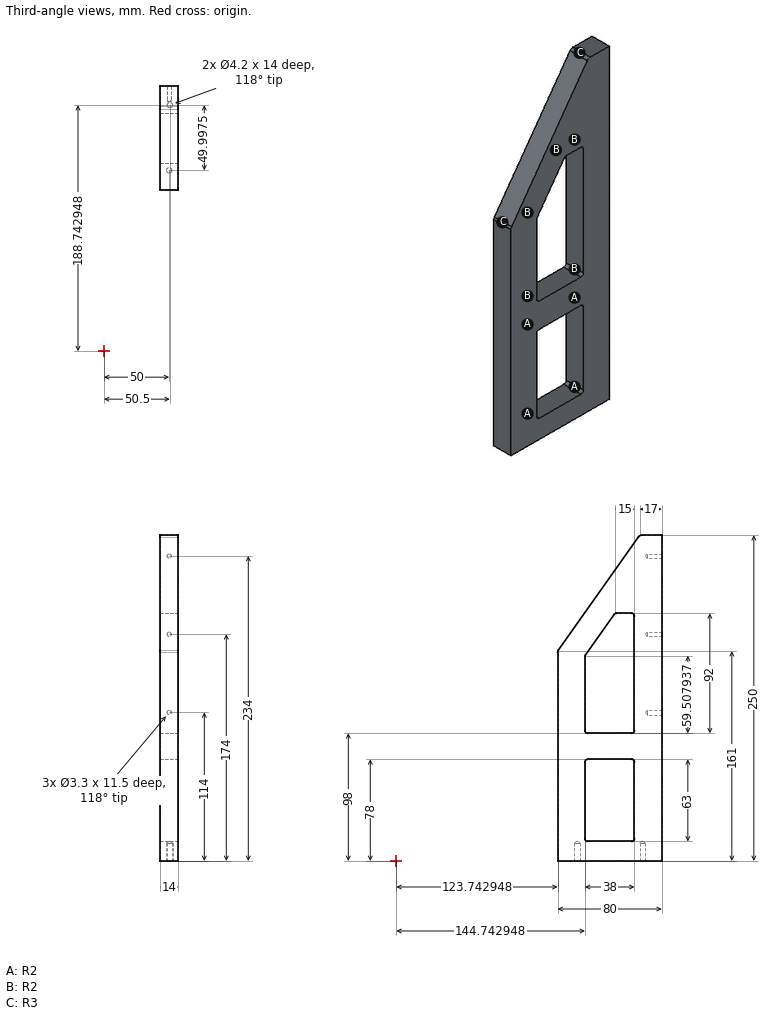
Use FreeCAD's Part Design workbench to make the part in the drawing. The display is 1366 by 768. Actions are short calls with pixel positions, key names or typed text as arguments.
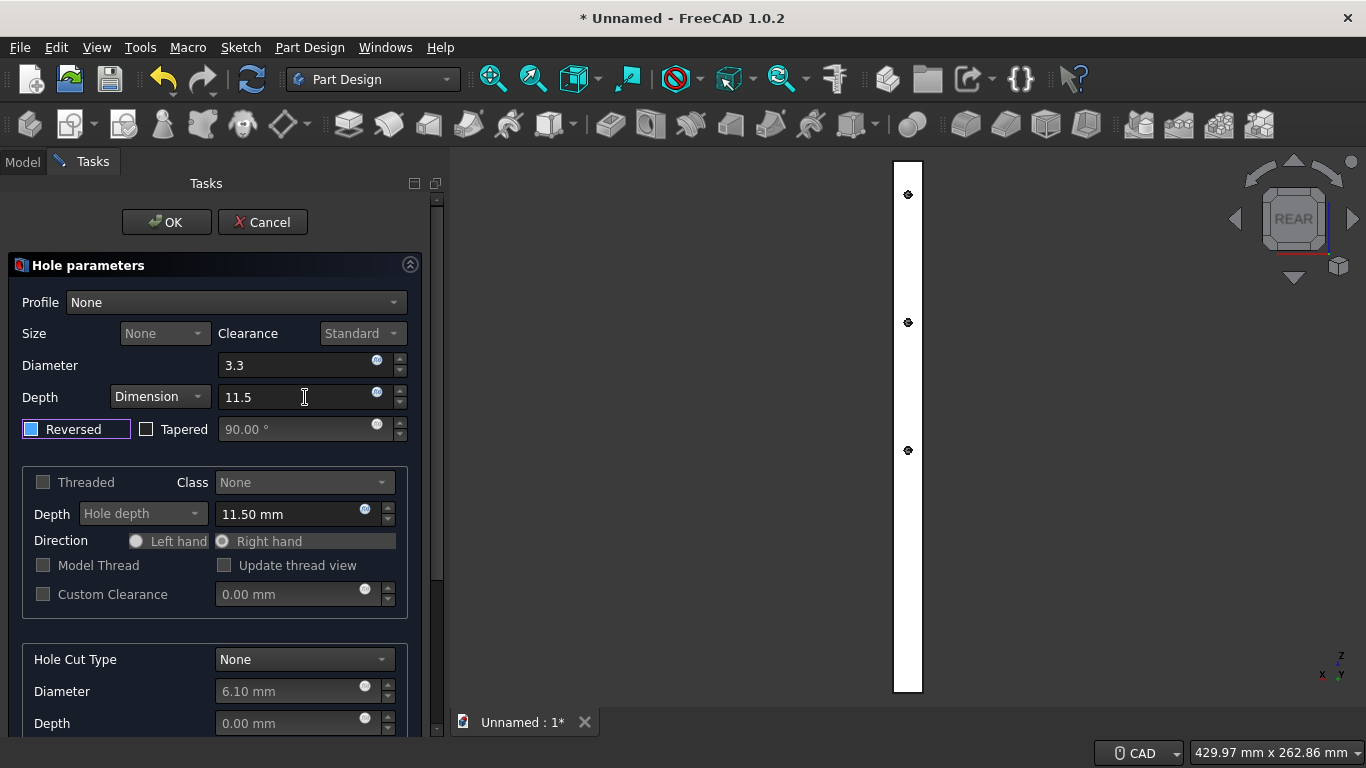
click(167, 222)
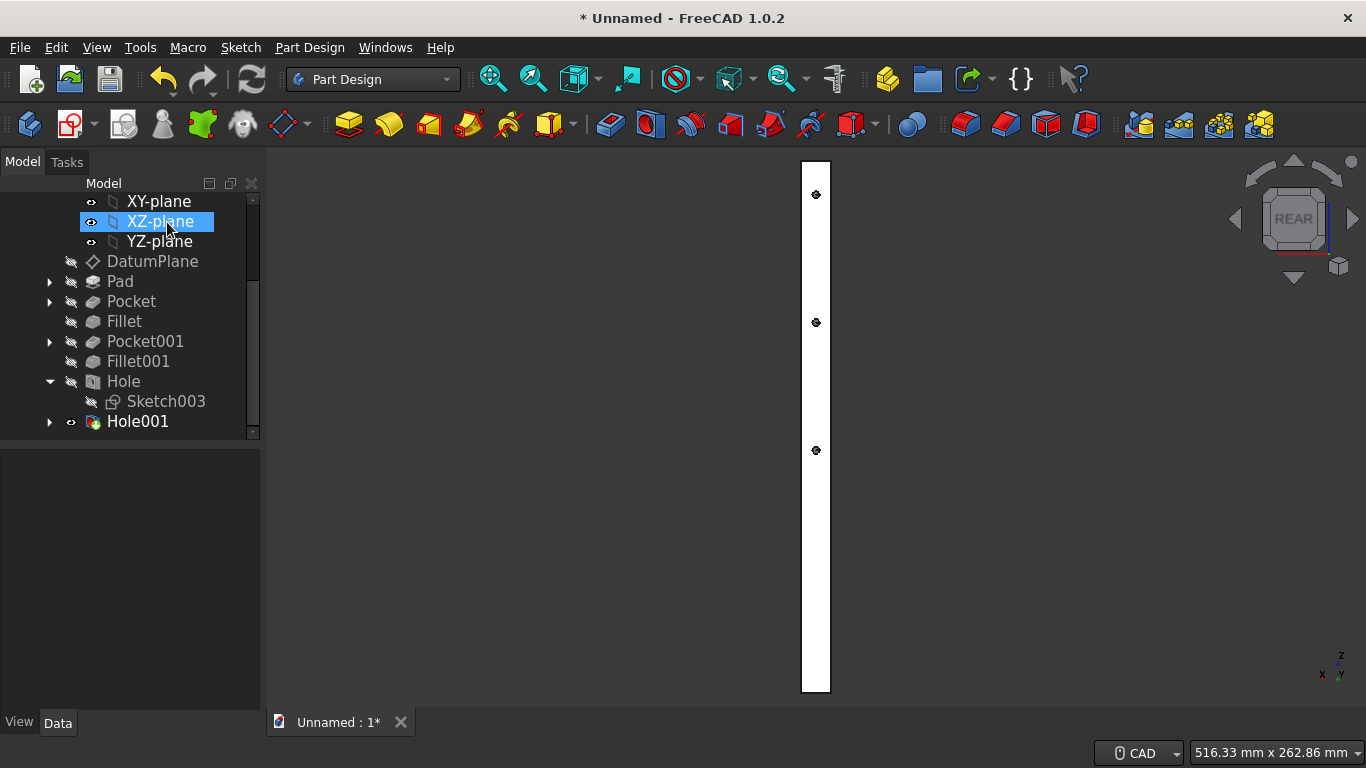
key(0)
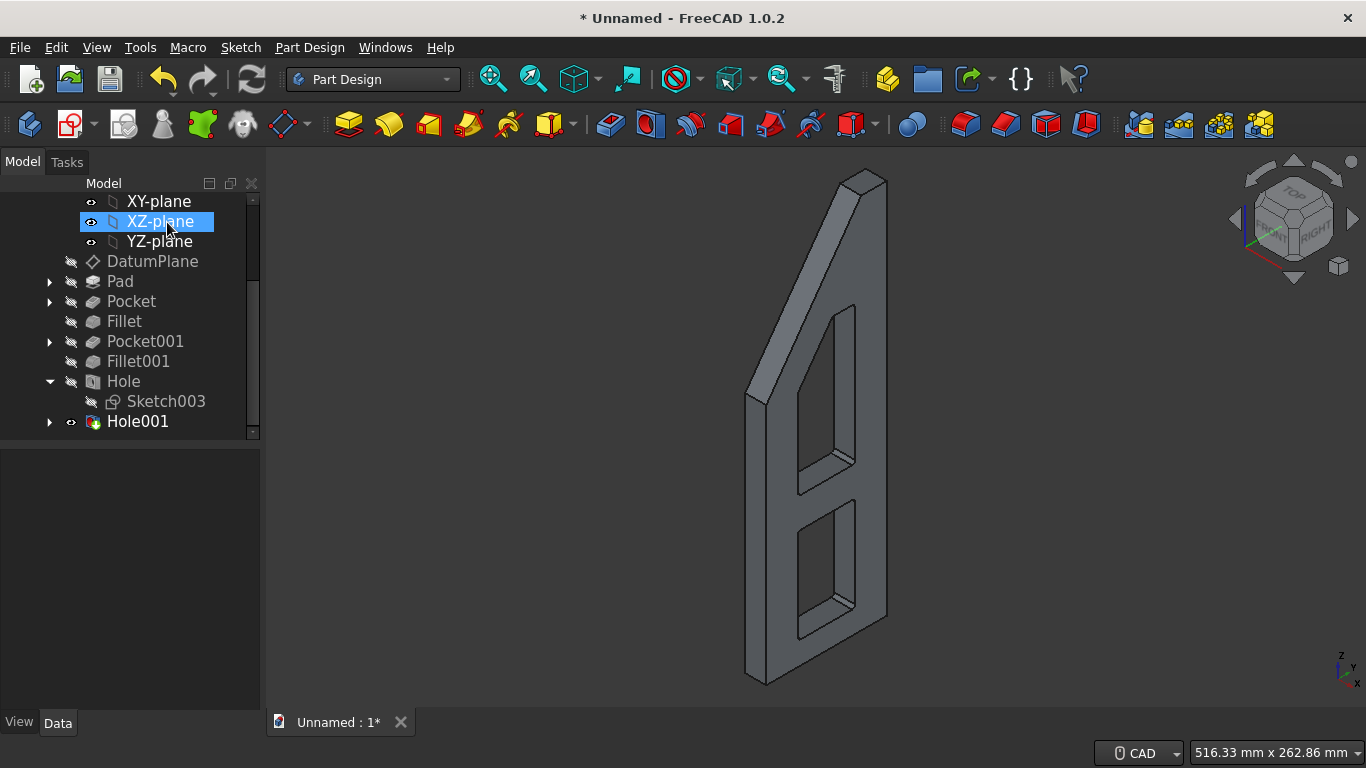
click(851, 189)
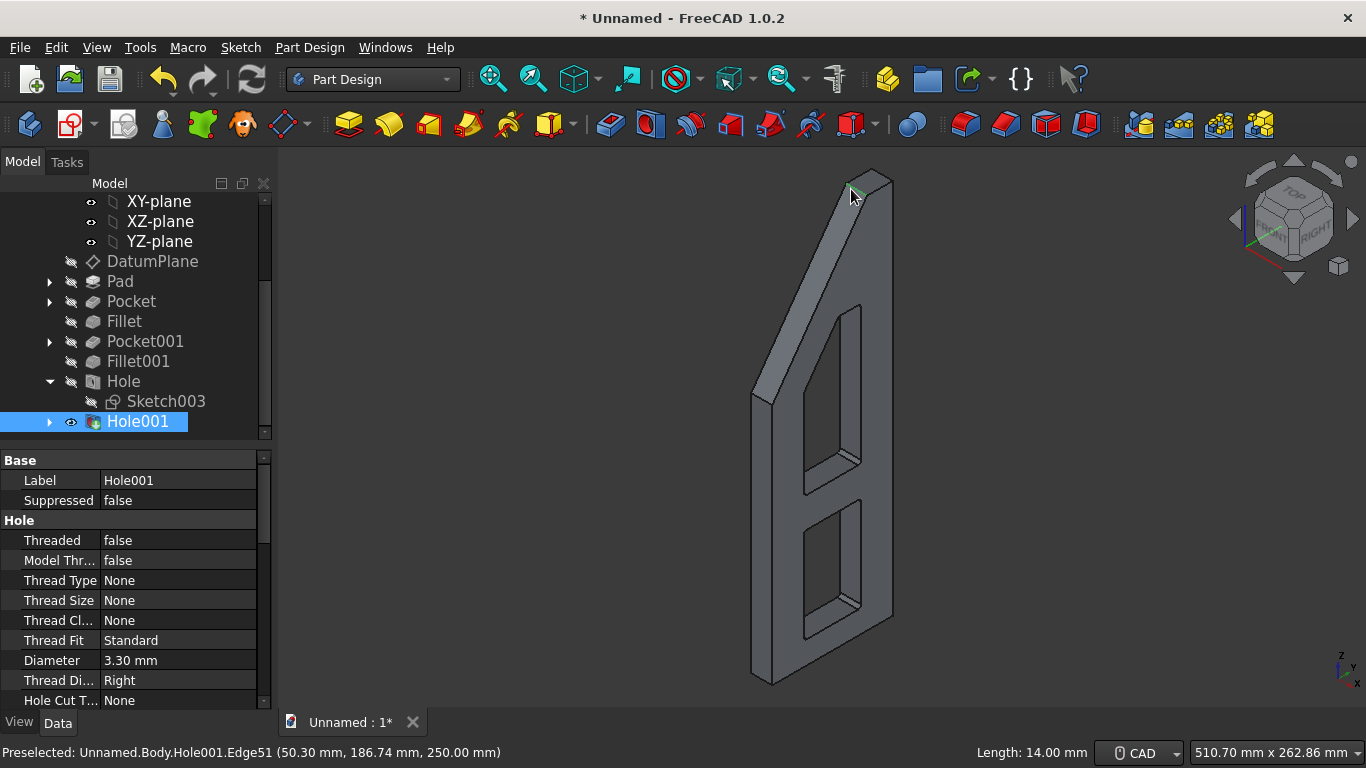
key(2)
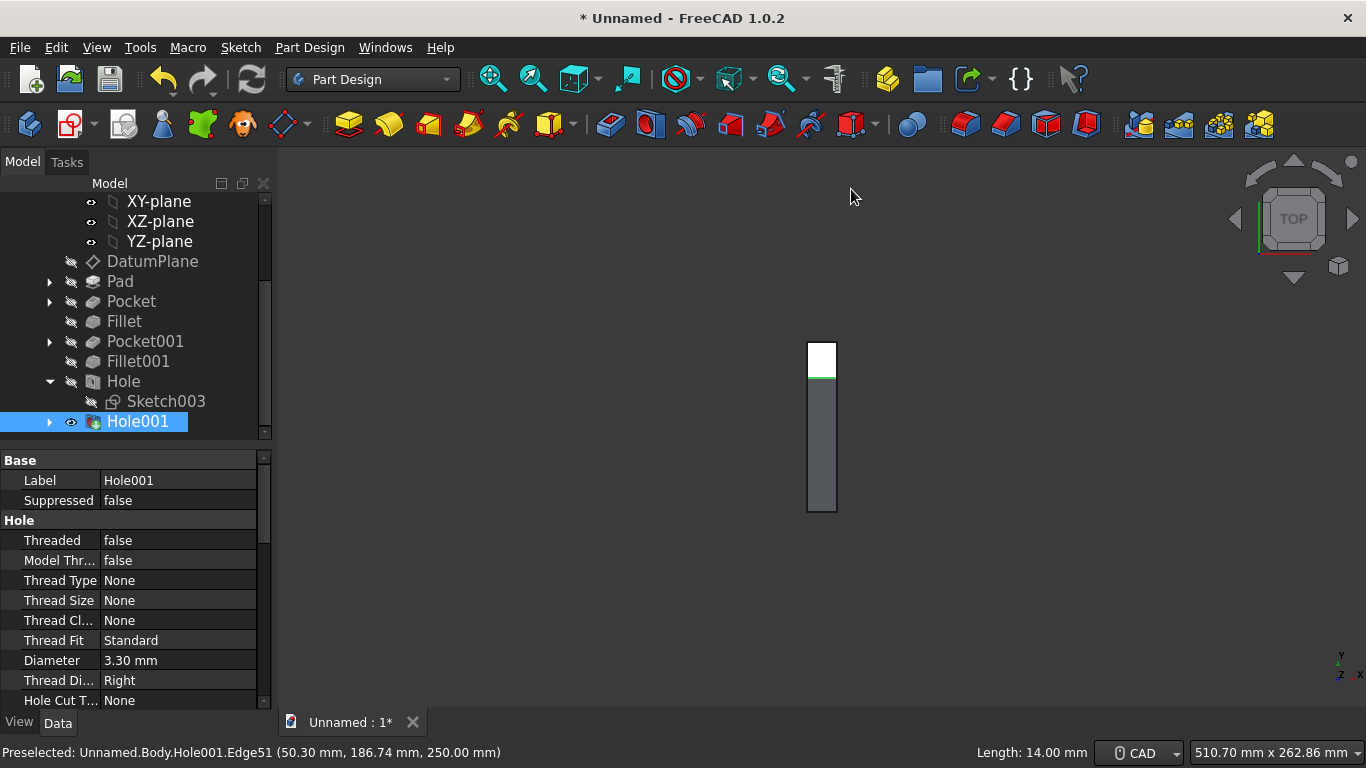
click(494, 80)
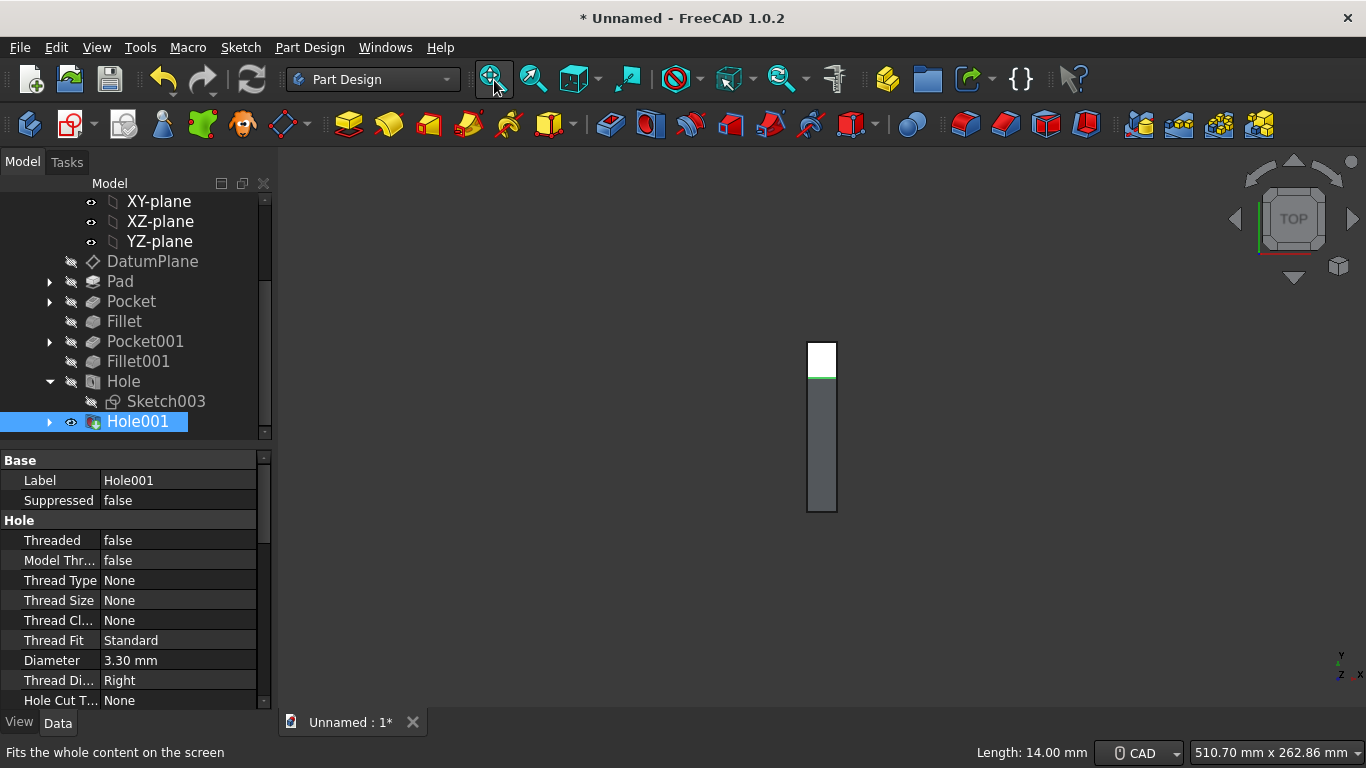
key(1)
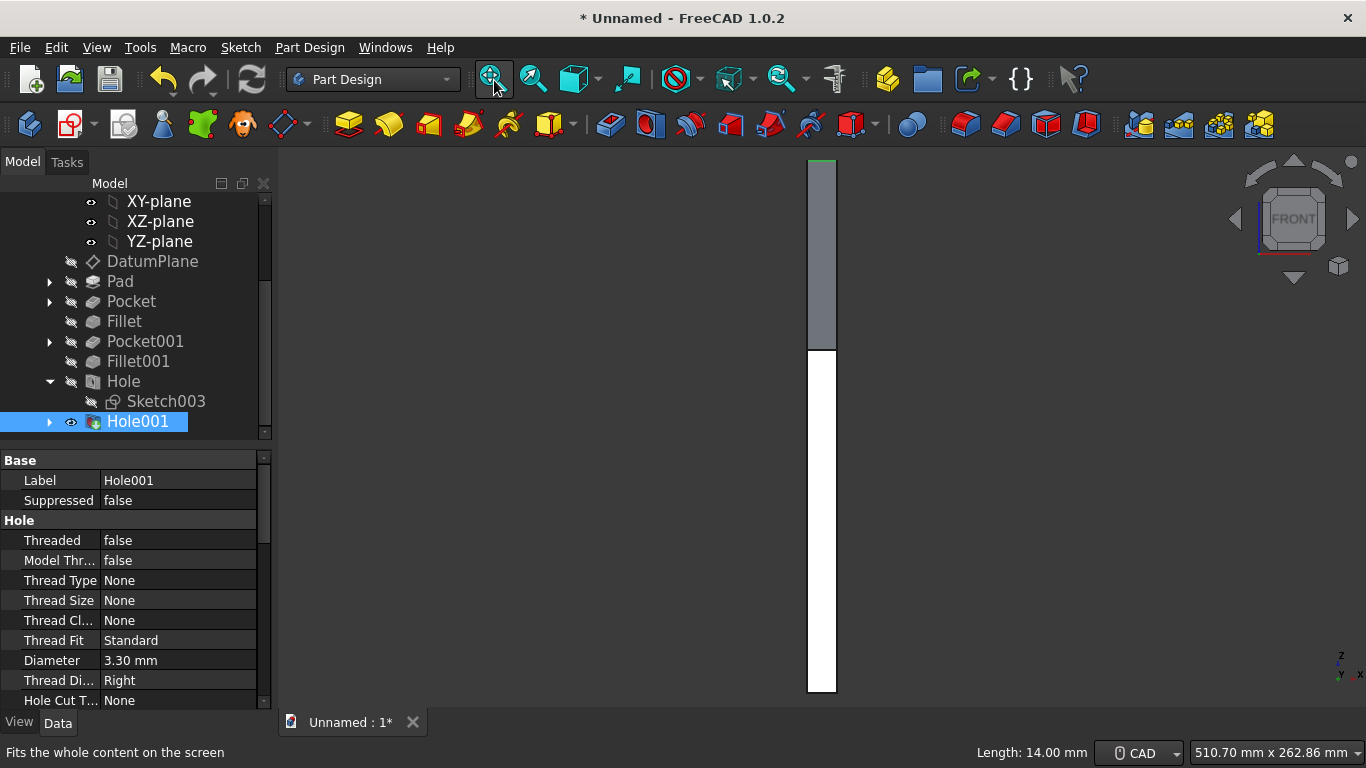
click(822, 349, ctrl)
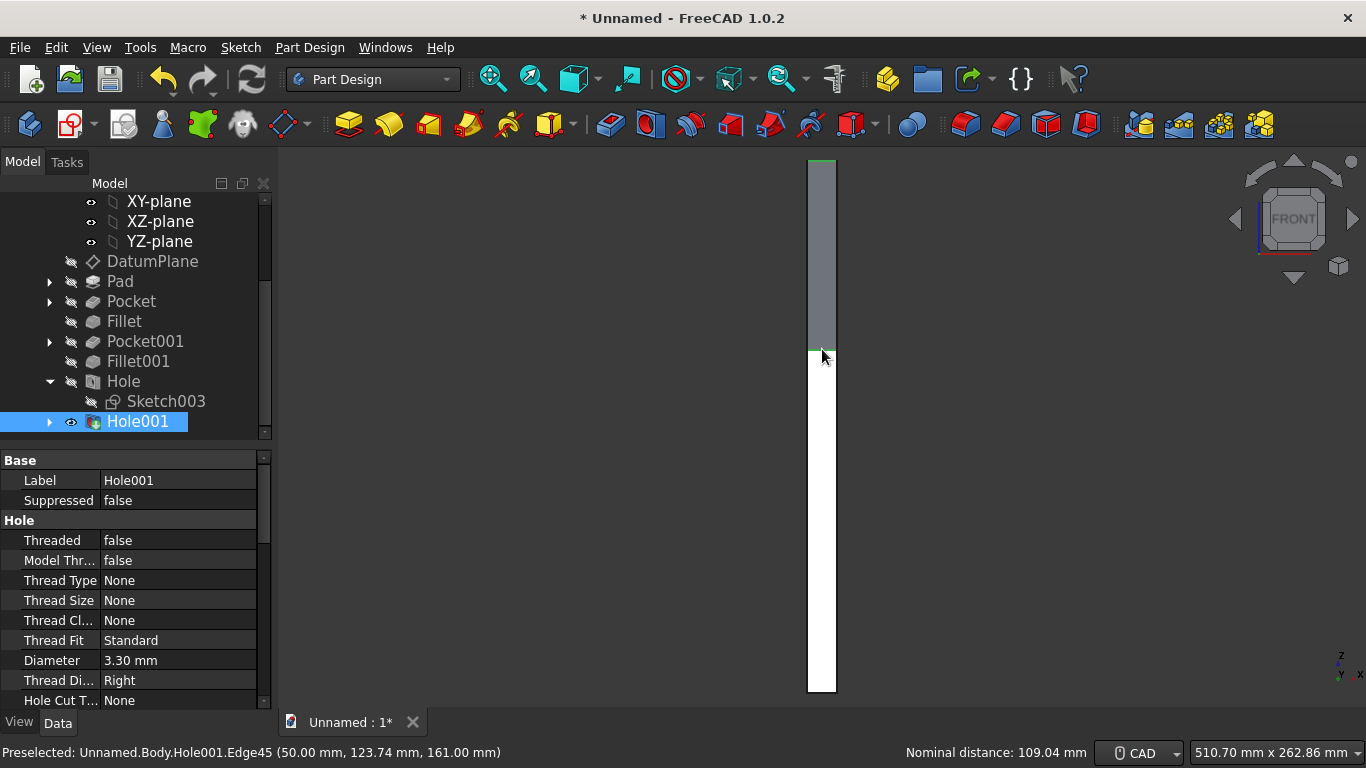
click(966, 124)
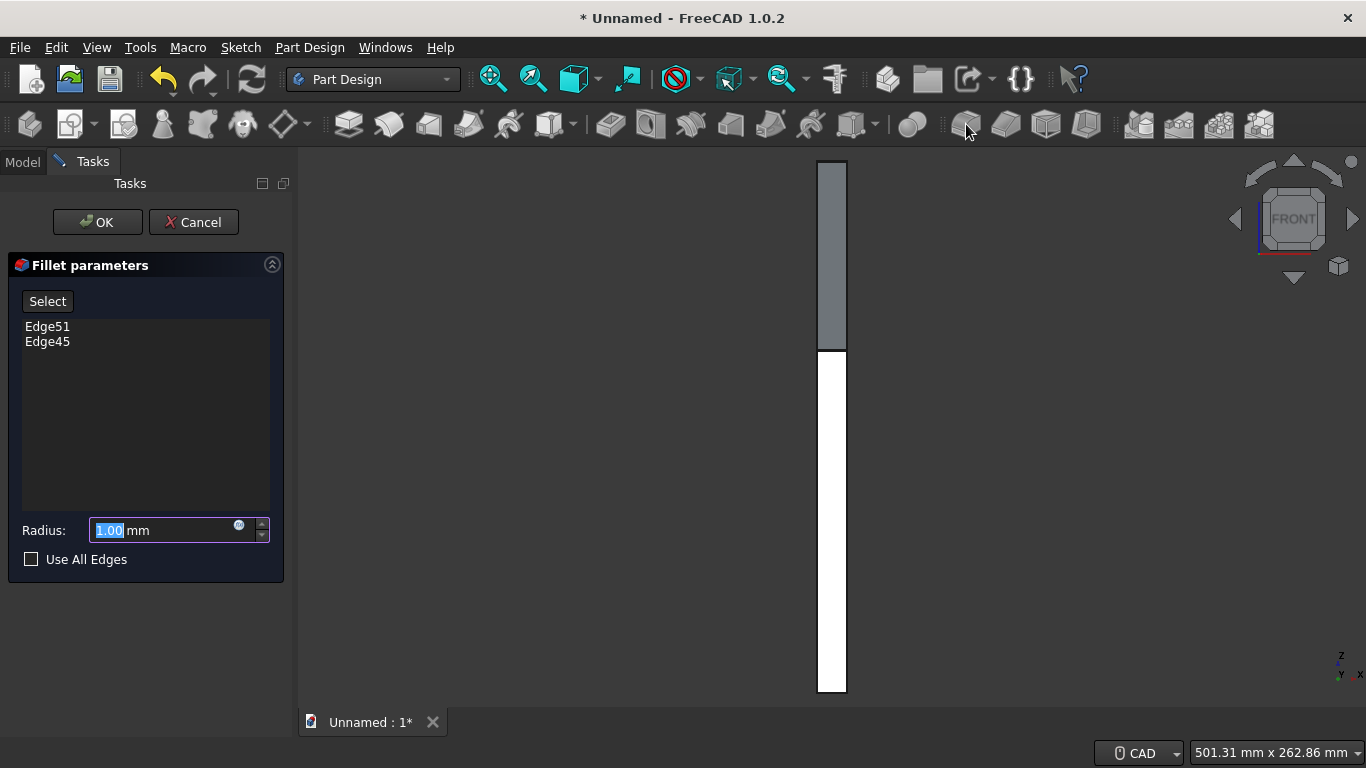
text(3)
key(Tab)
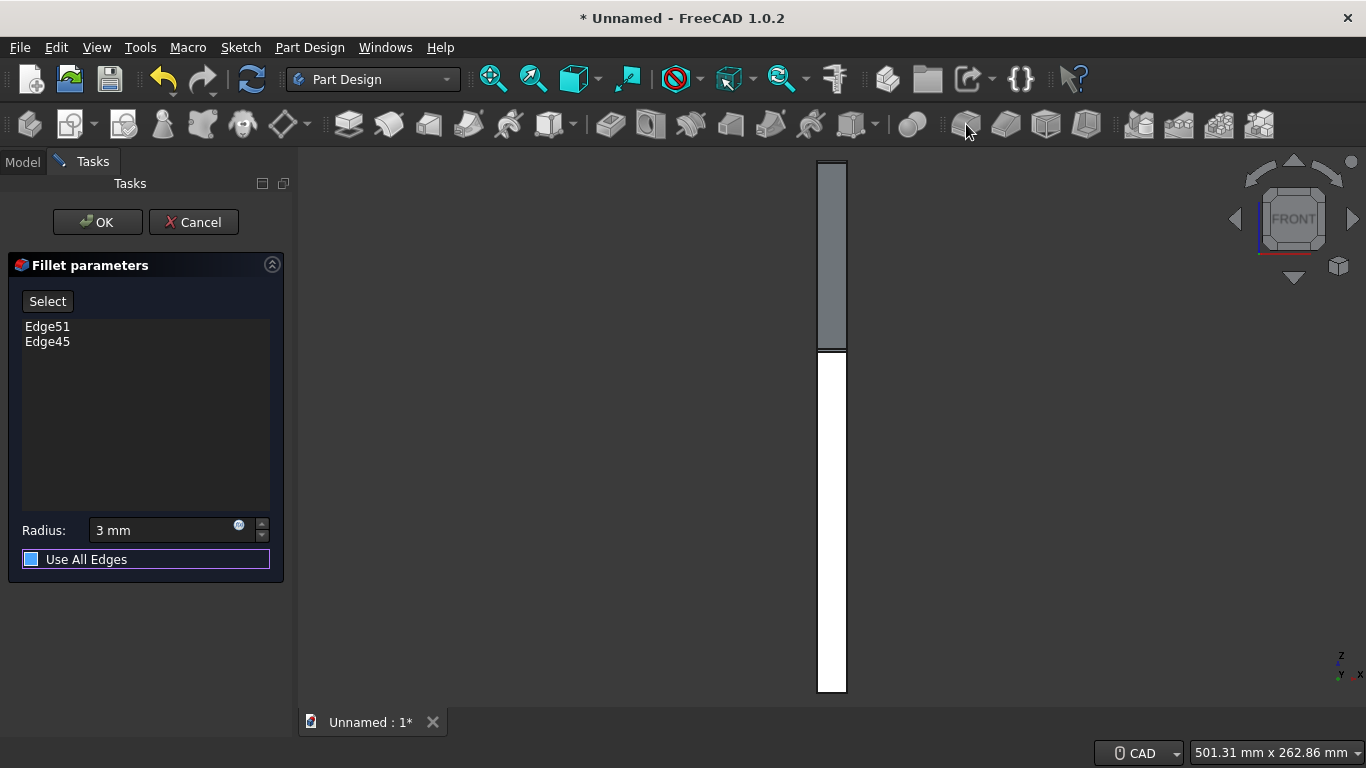
click(98, 222)